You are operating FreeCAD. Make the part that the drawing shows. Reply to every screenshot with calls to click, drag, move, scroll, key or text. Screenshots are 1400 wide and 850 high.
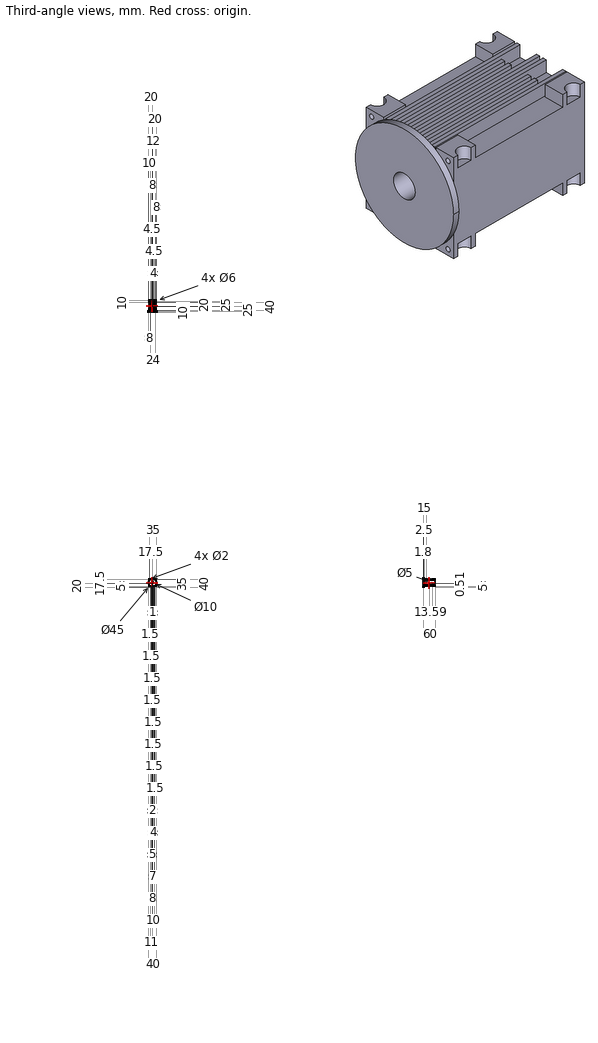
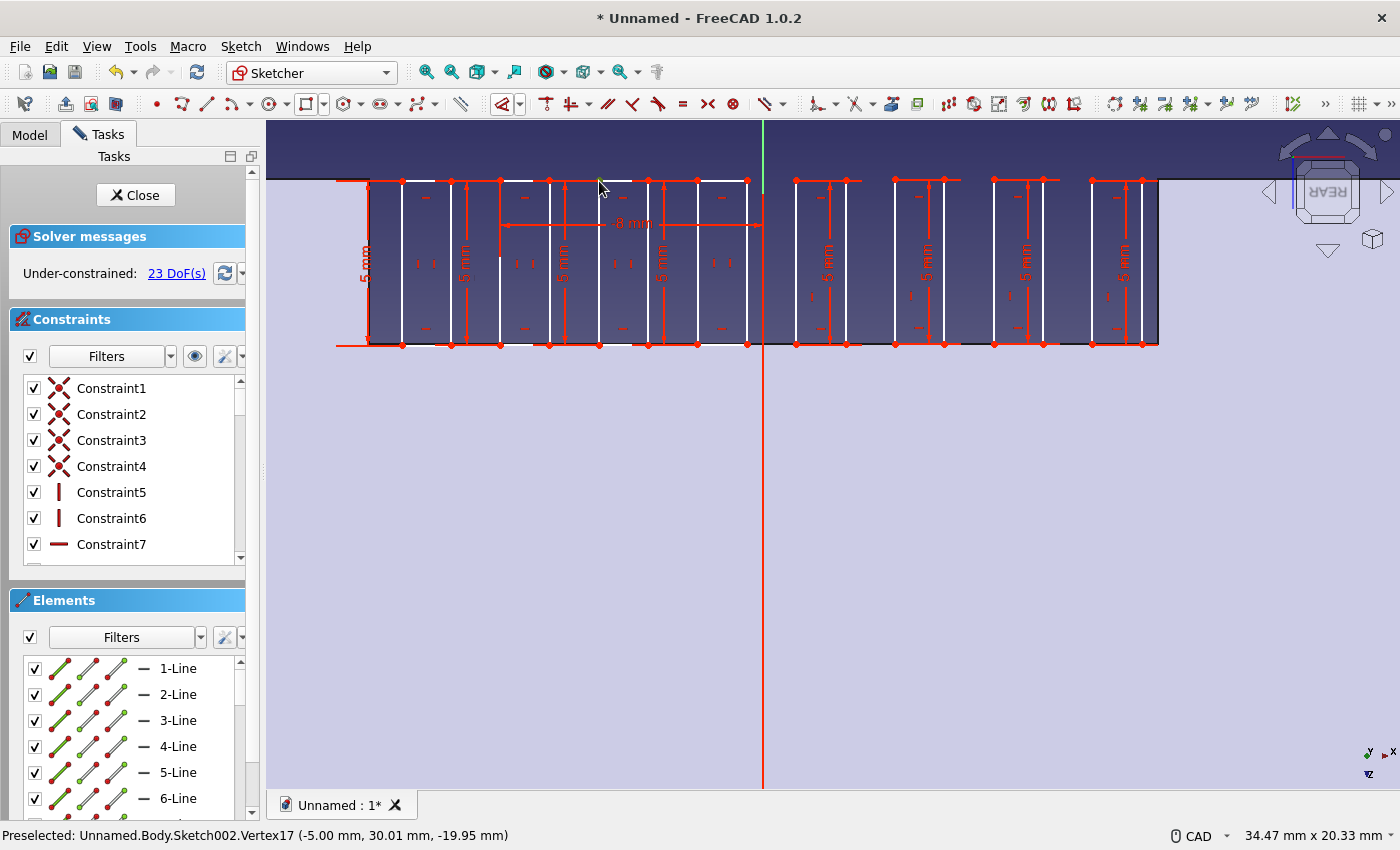
click(520, 104)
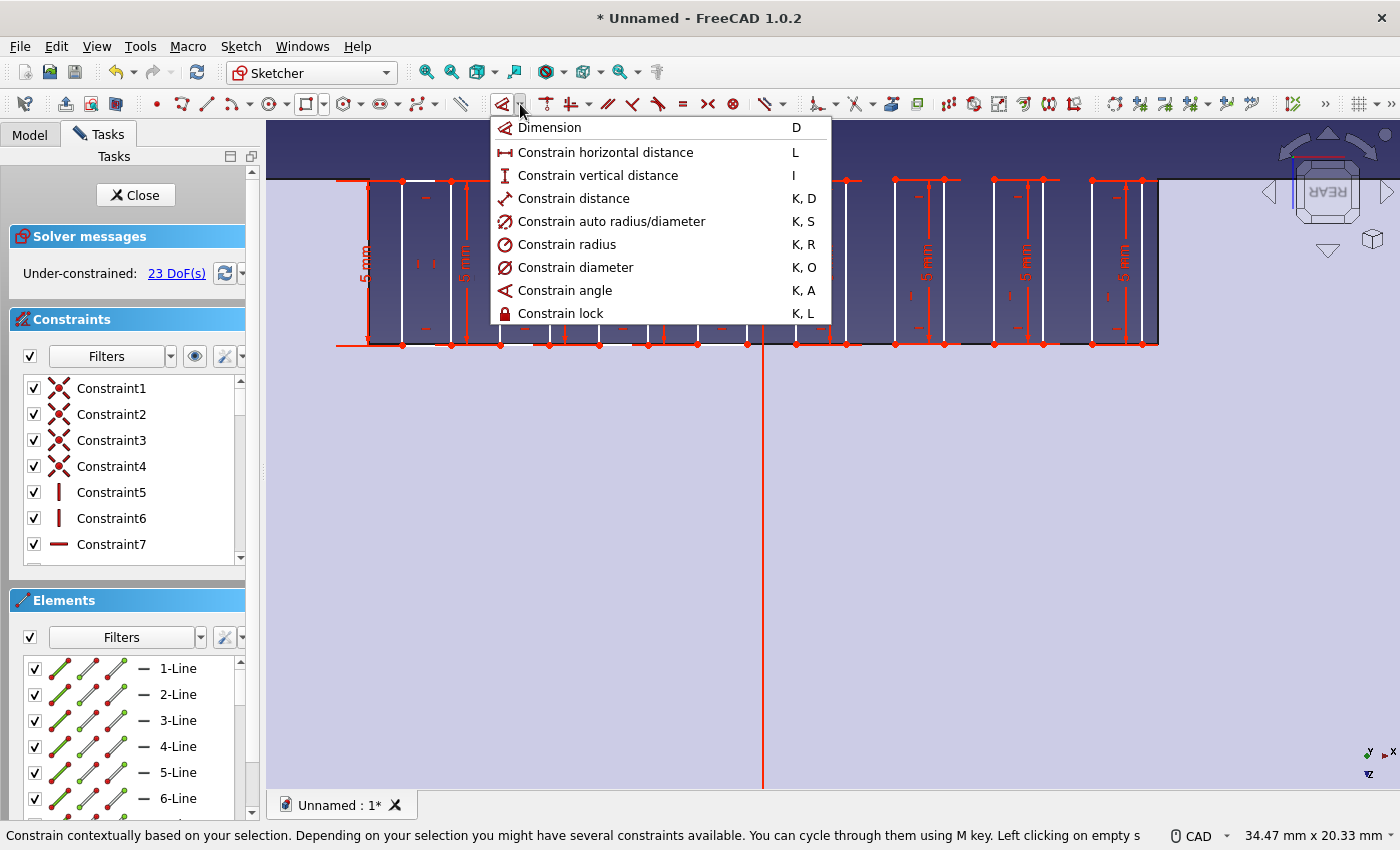
click(661, 152)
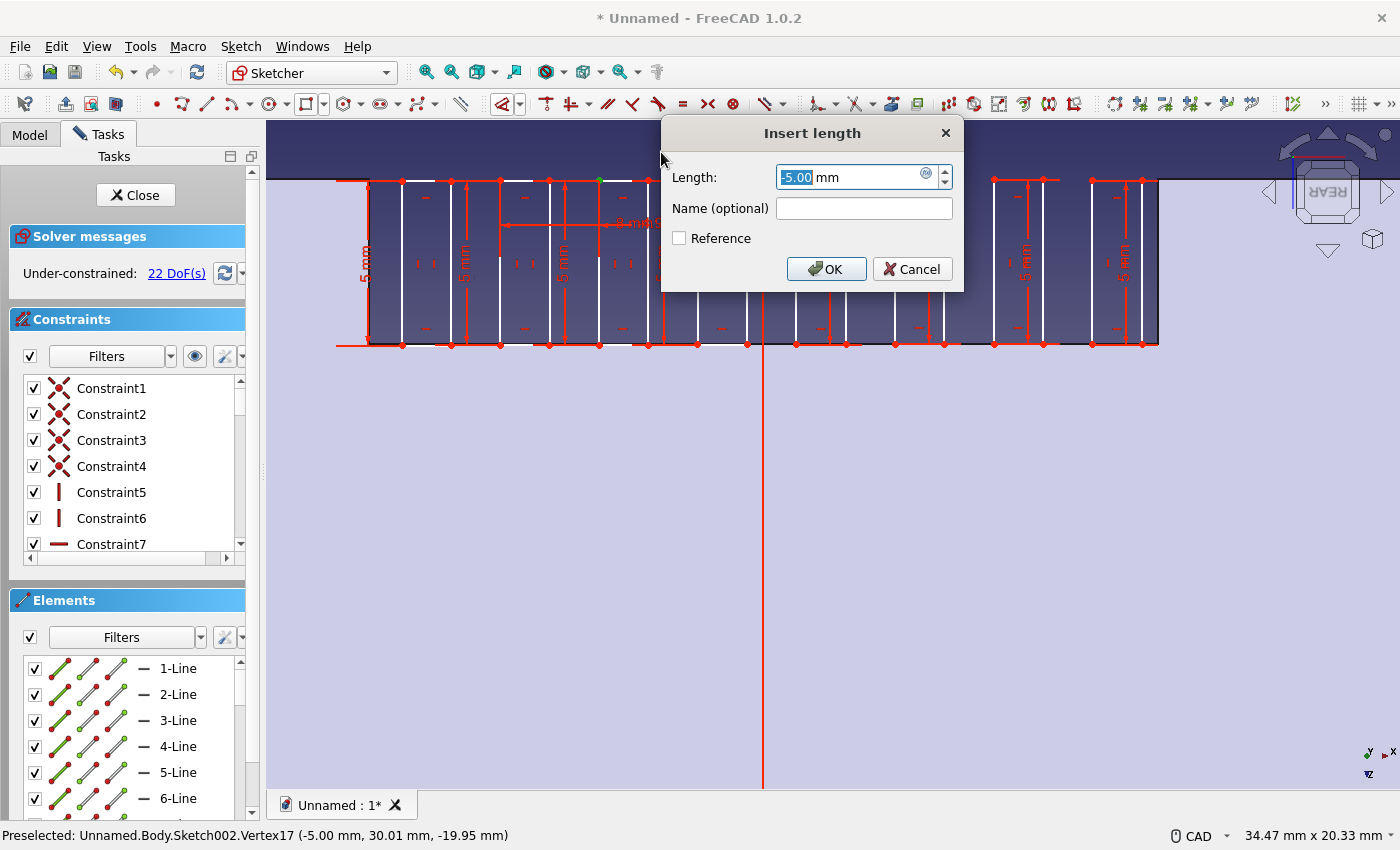
text(-5)
key(Return)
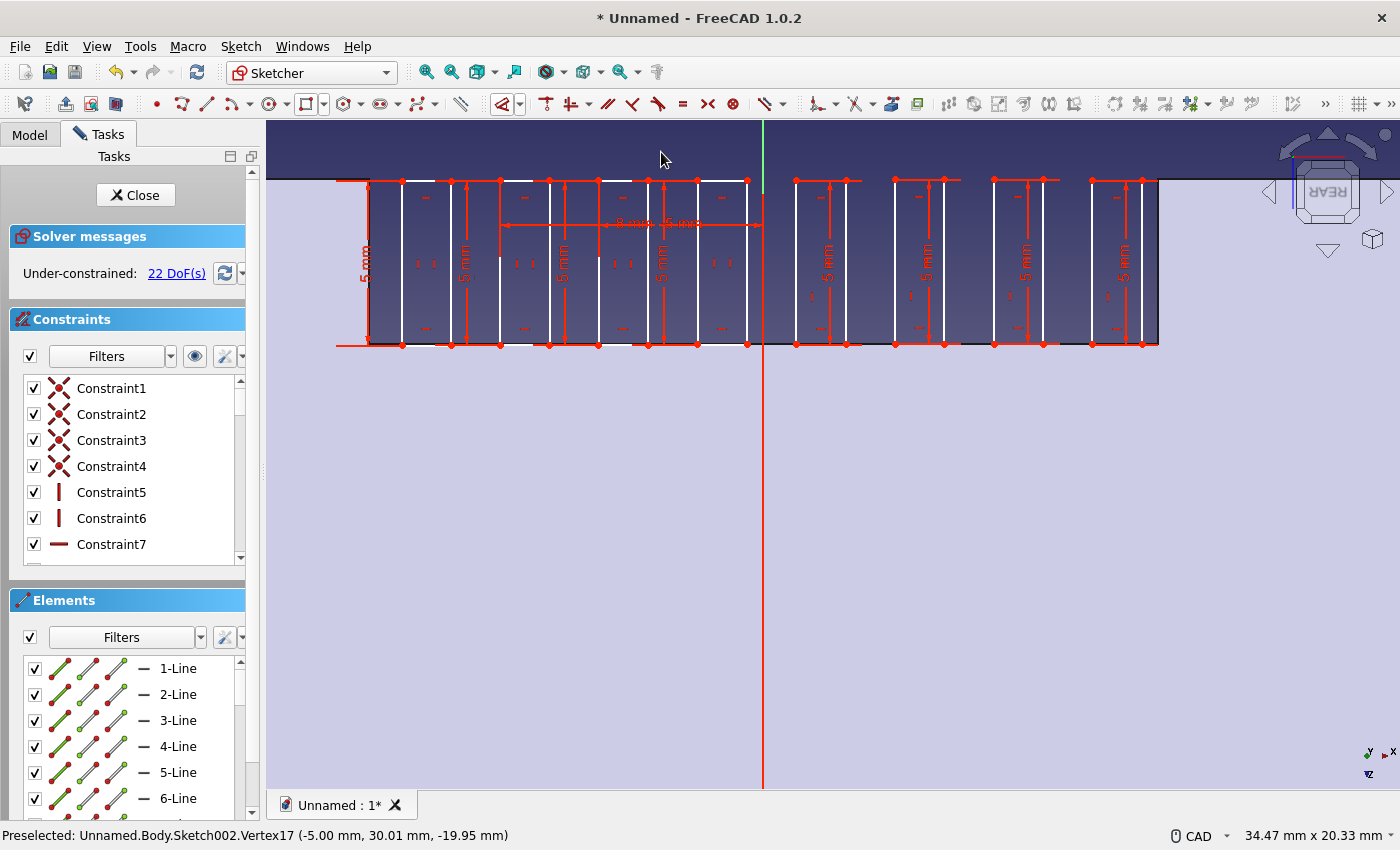
click(698, 181)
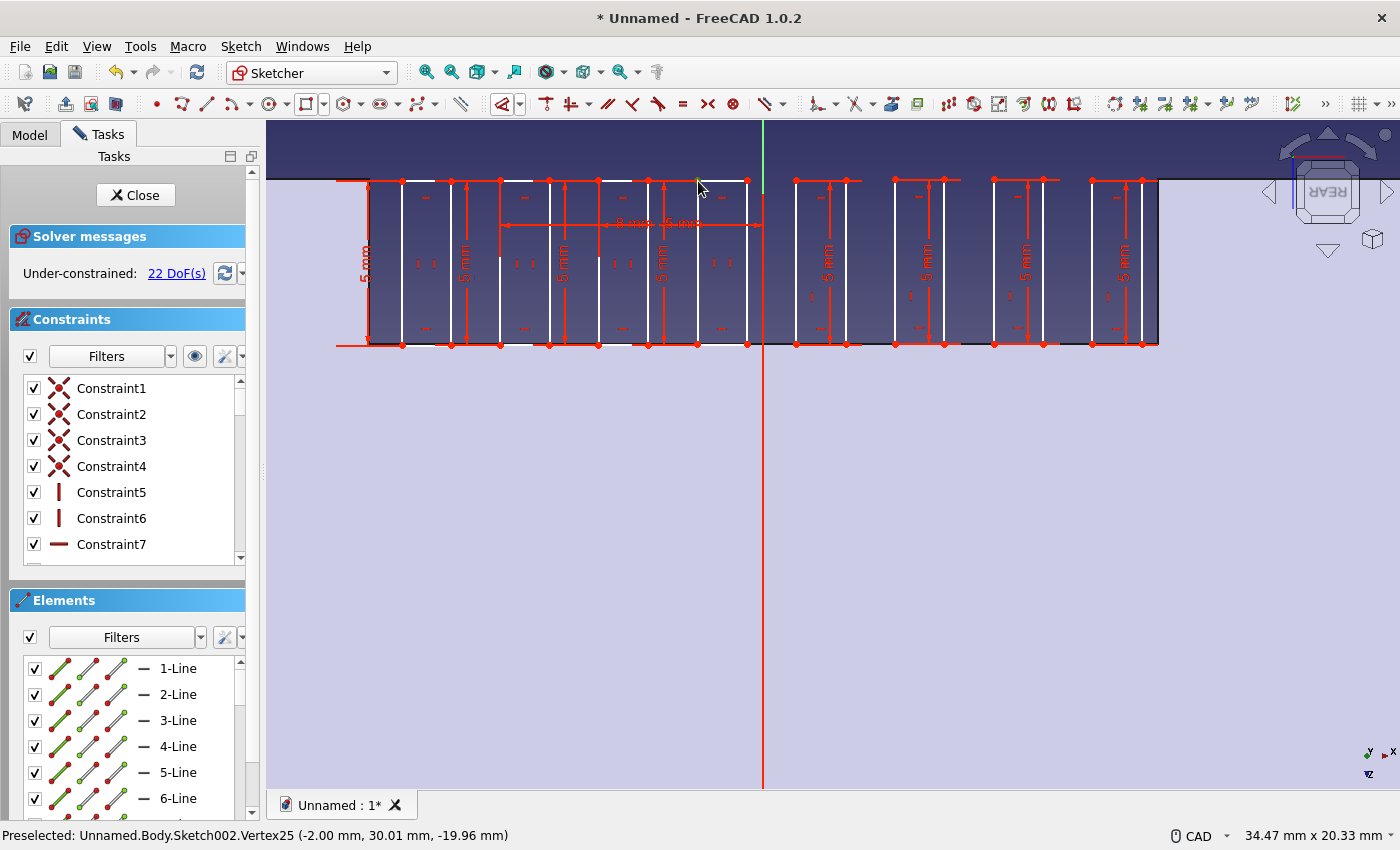
key(l)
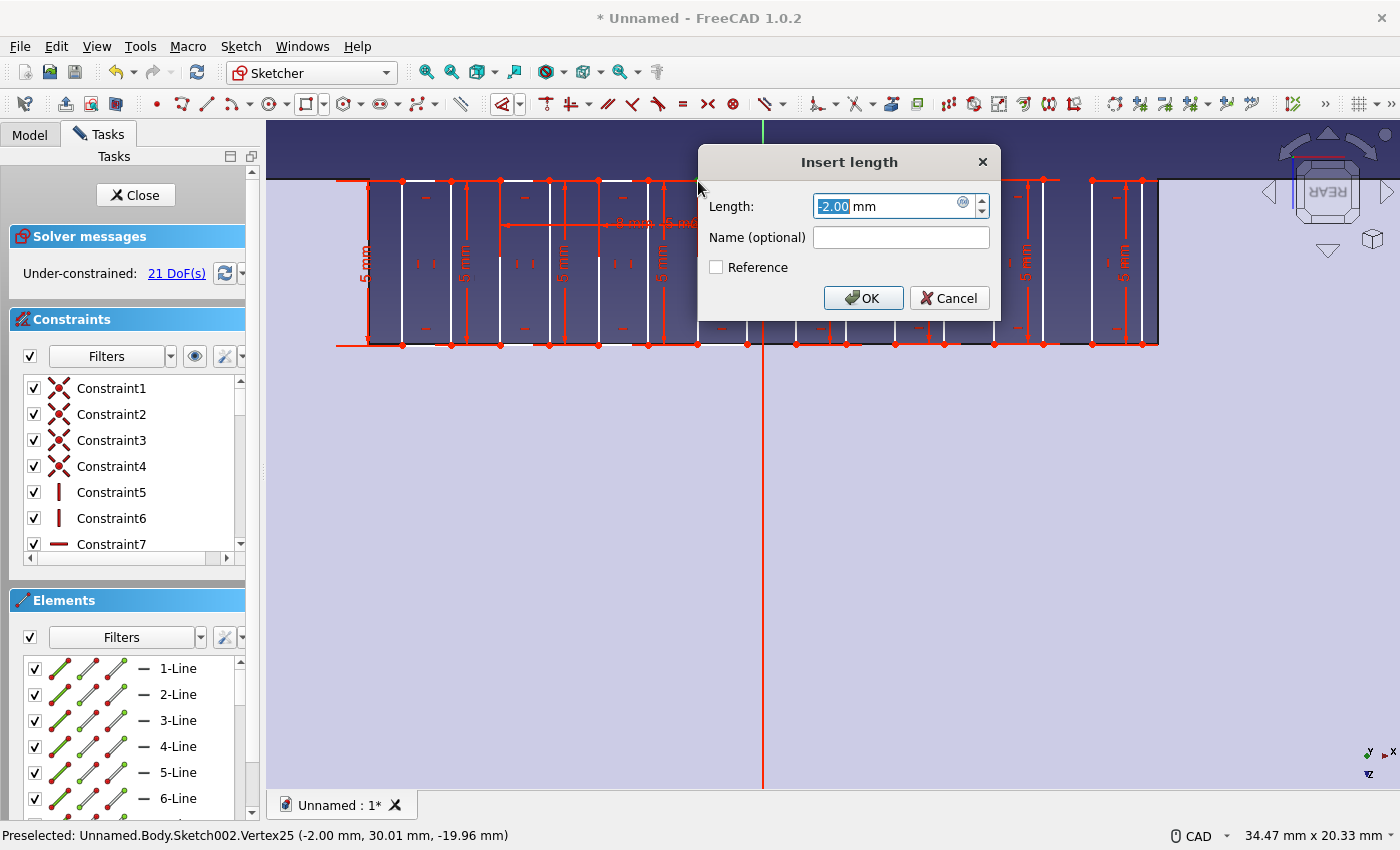
text(-2)
key(Return)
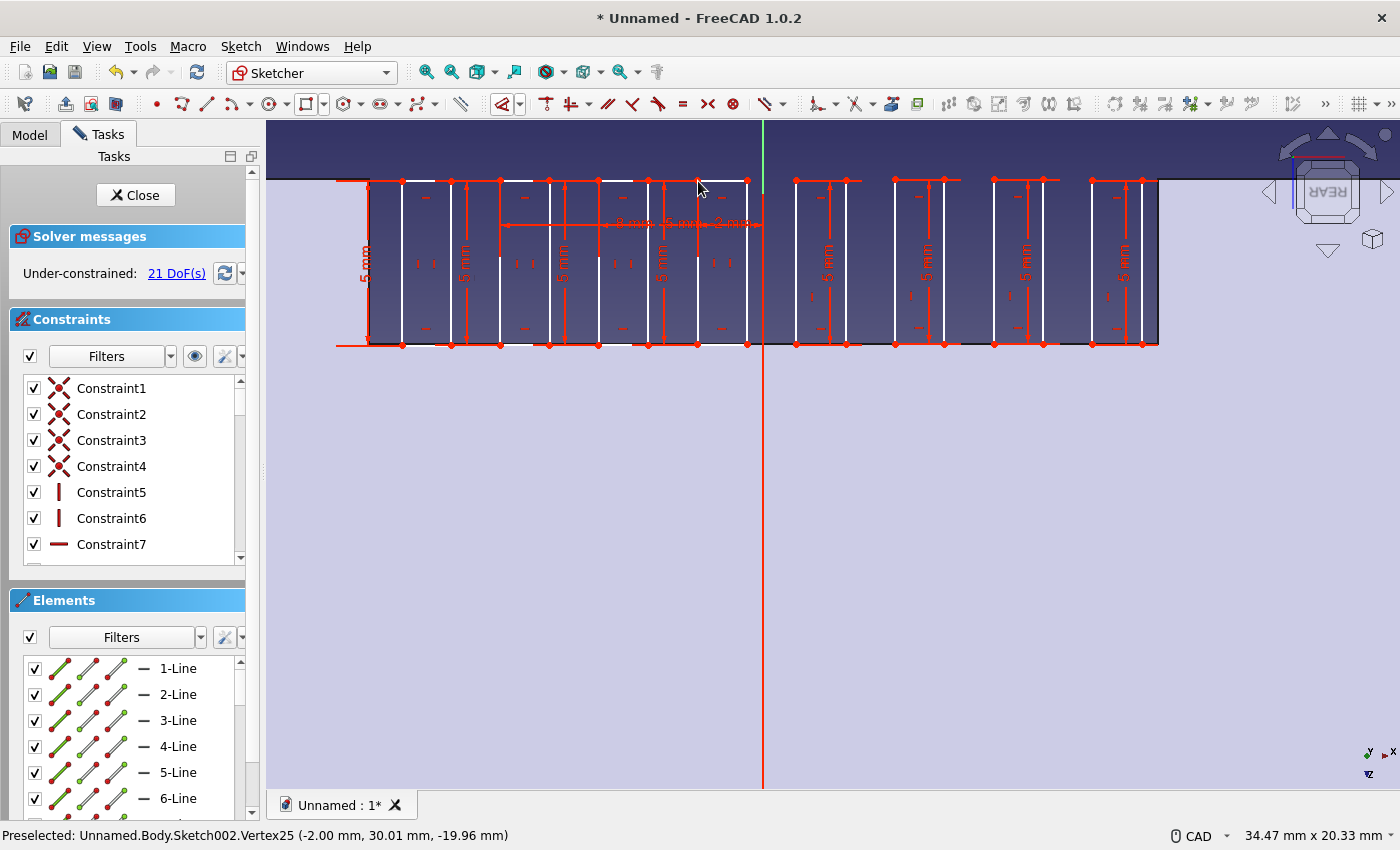
click(796, 181)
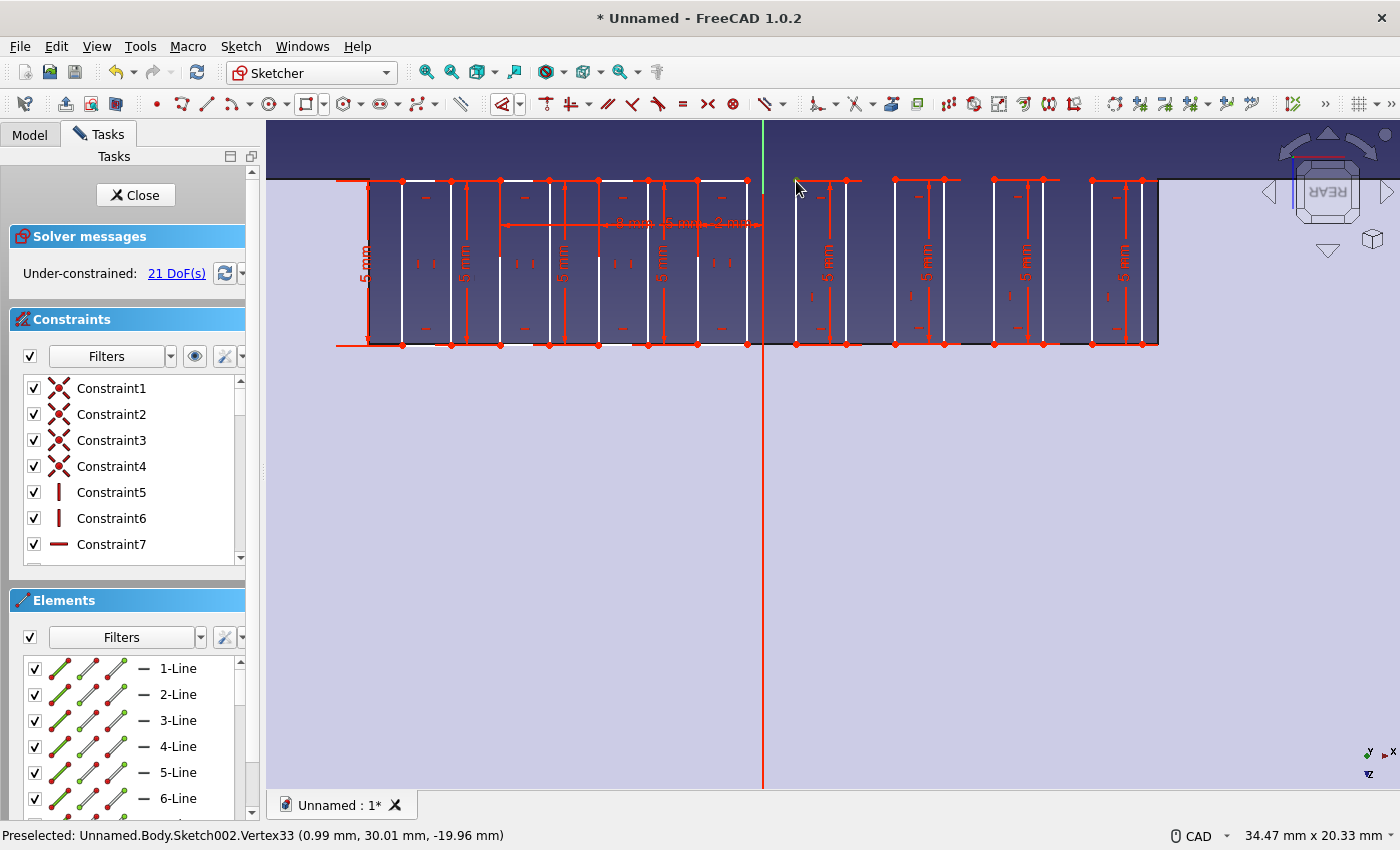
click(520, 104)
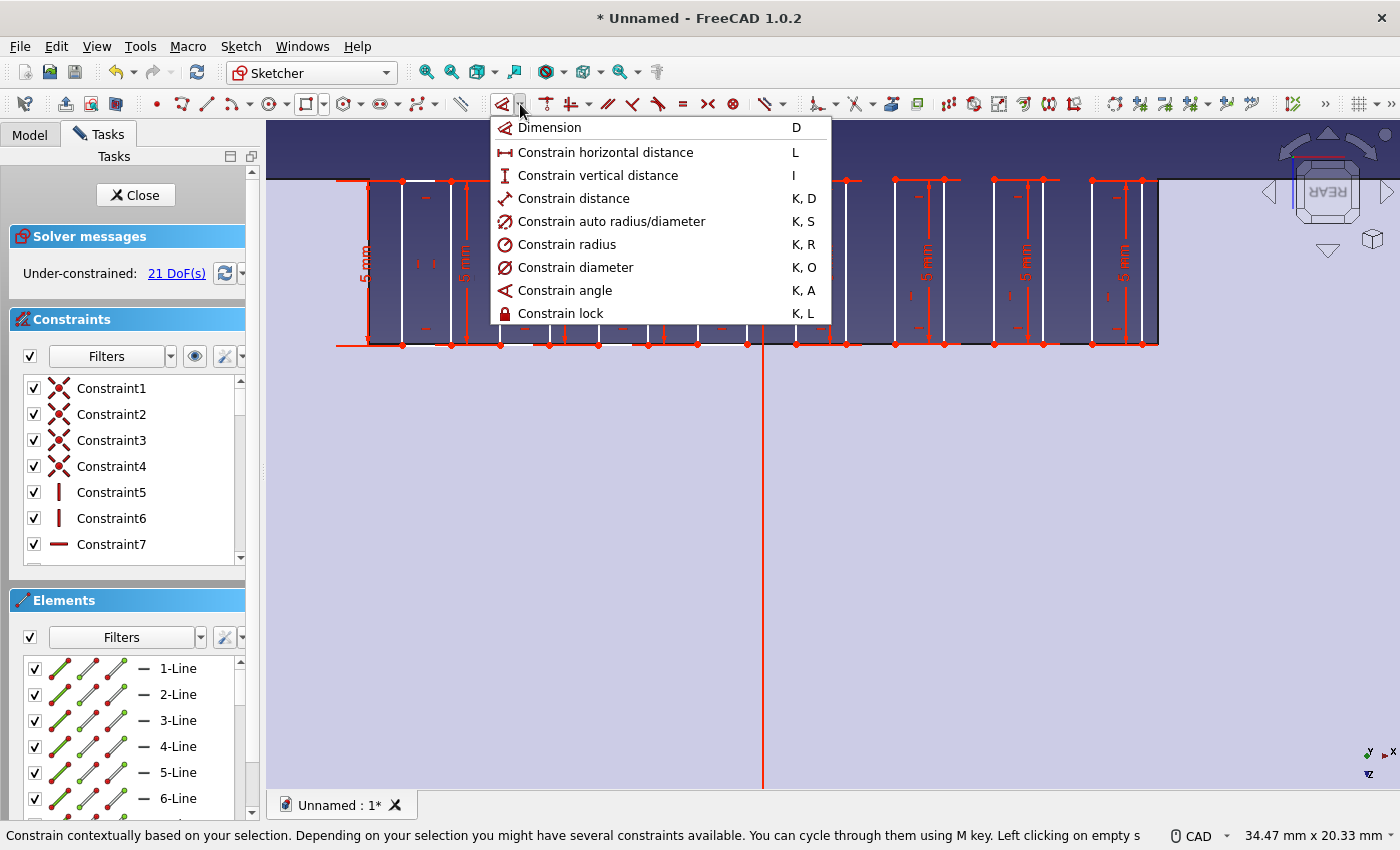
click(661, 152)